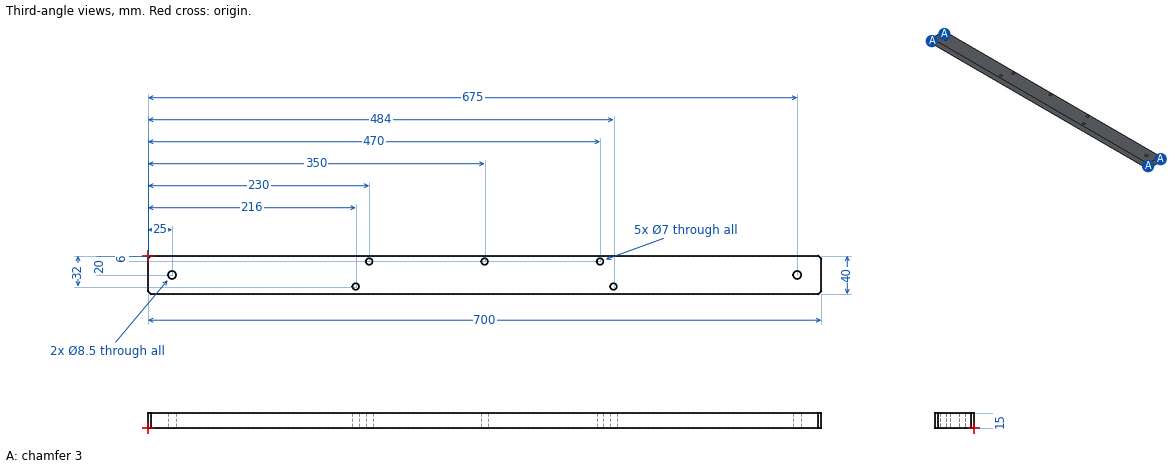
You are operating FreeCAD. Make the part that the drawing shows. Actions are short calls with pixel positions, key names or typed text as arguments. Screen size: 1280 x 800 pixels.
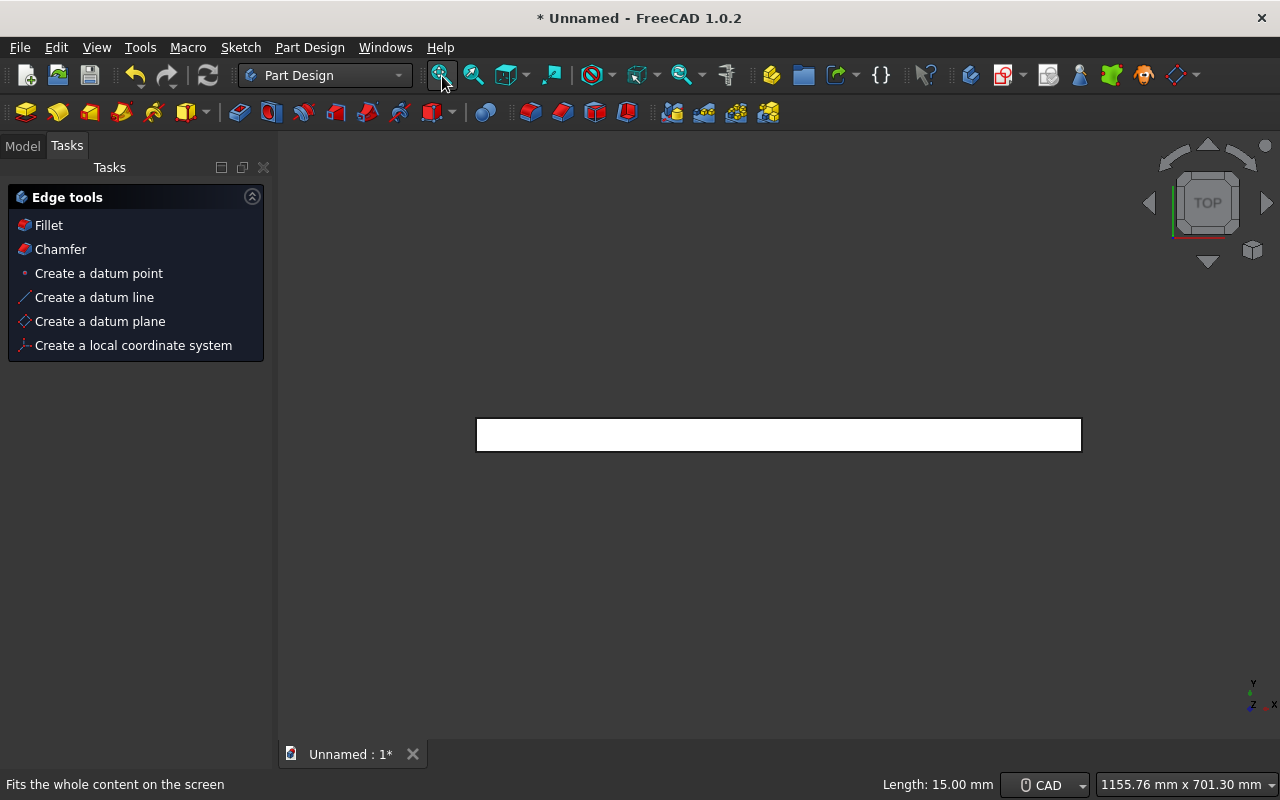
scroll(476, 417, up, 6)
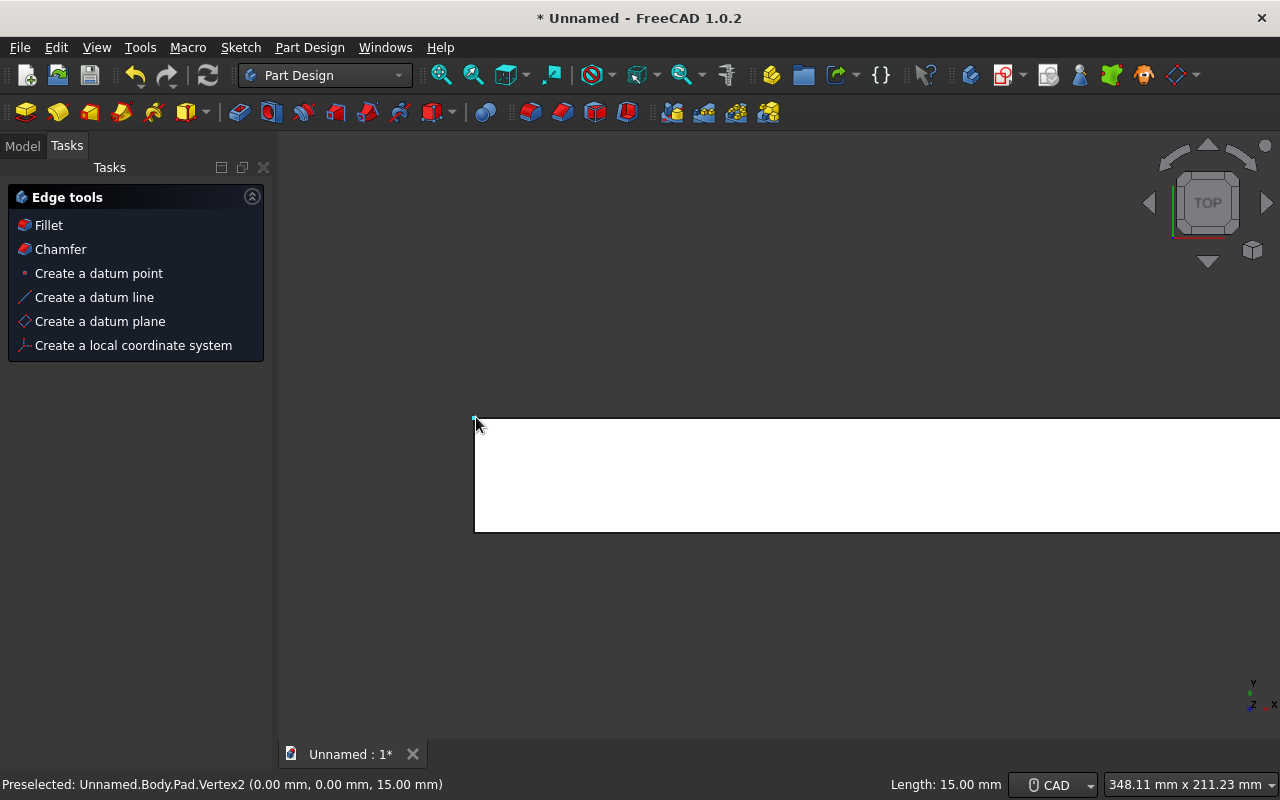
click(442, 76)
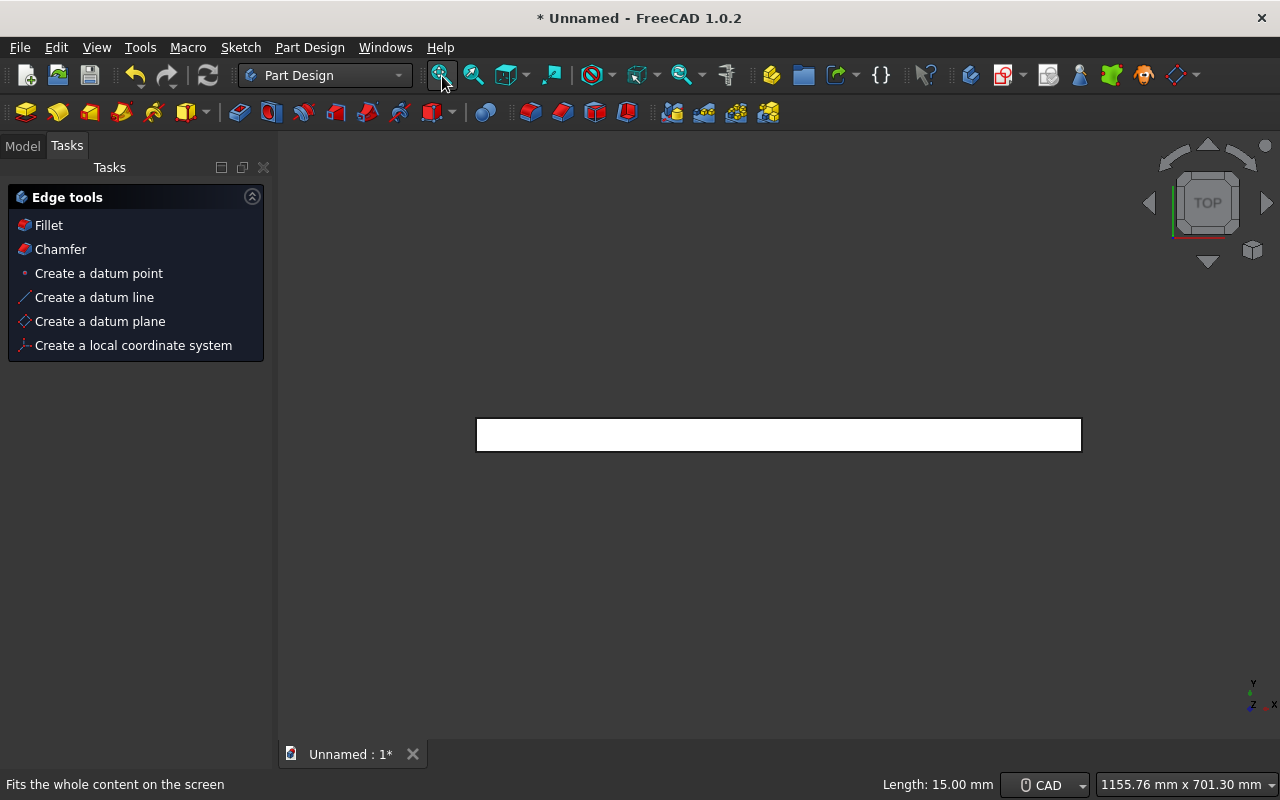
key(1)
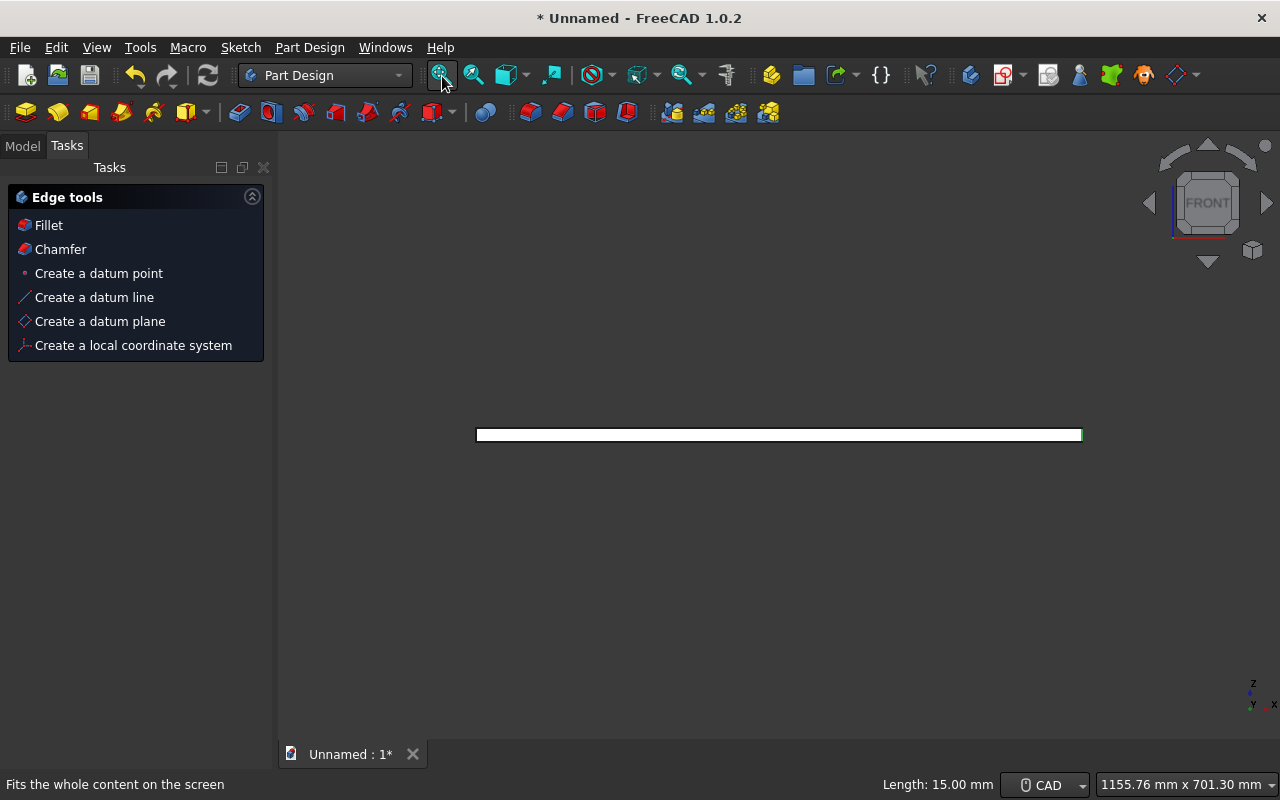
click(476, 434, ctrl)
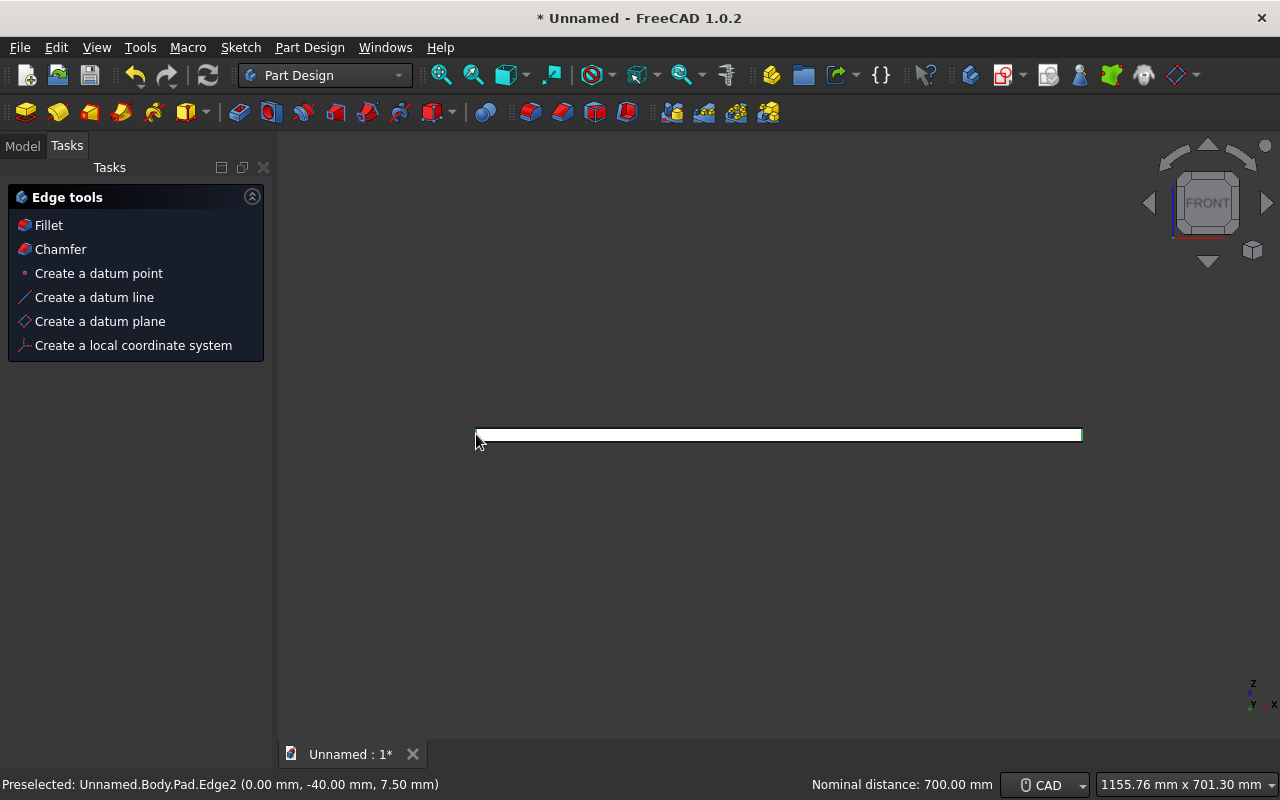
scroll(476, 434, up, 6)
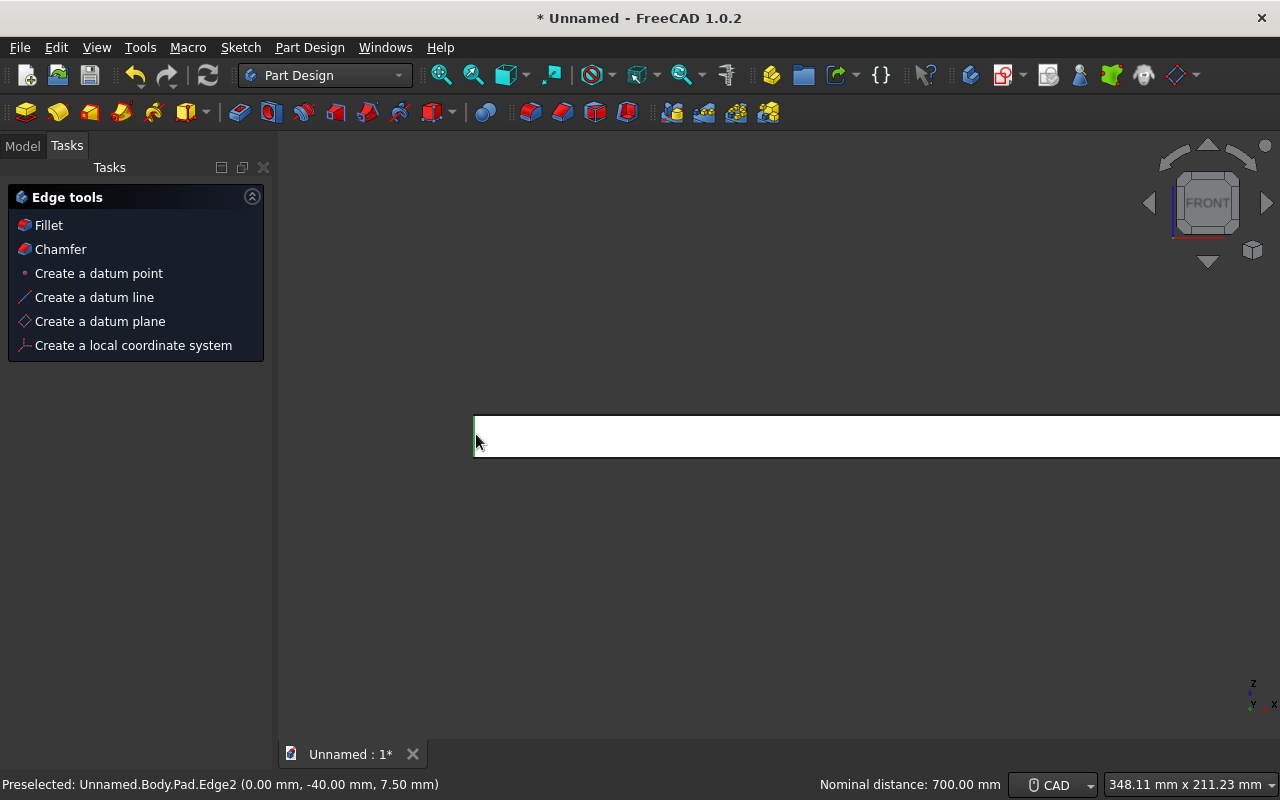
click(442, 76)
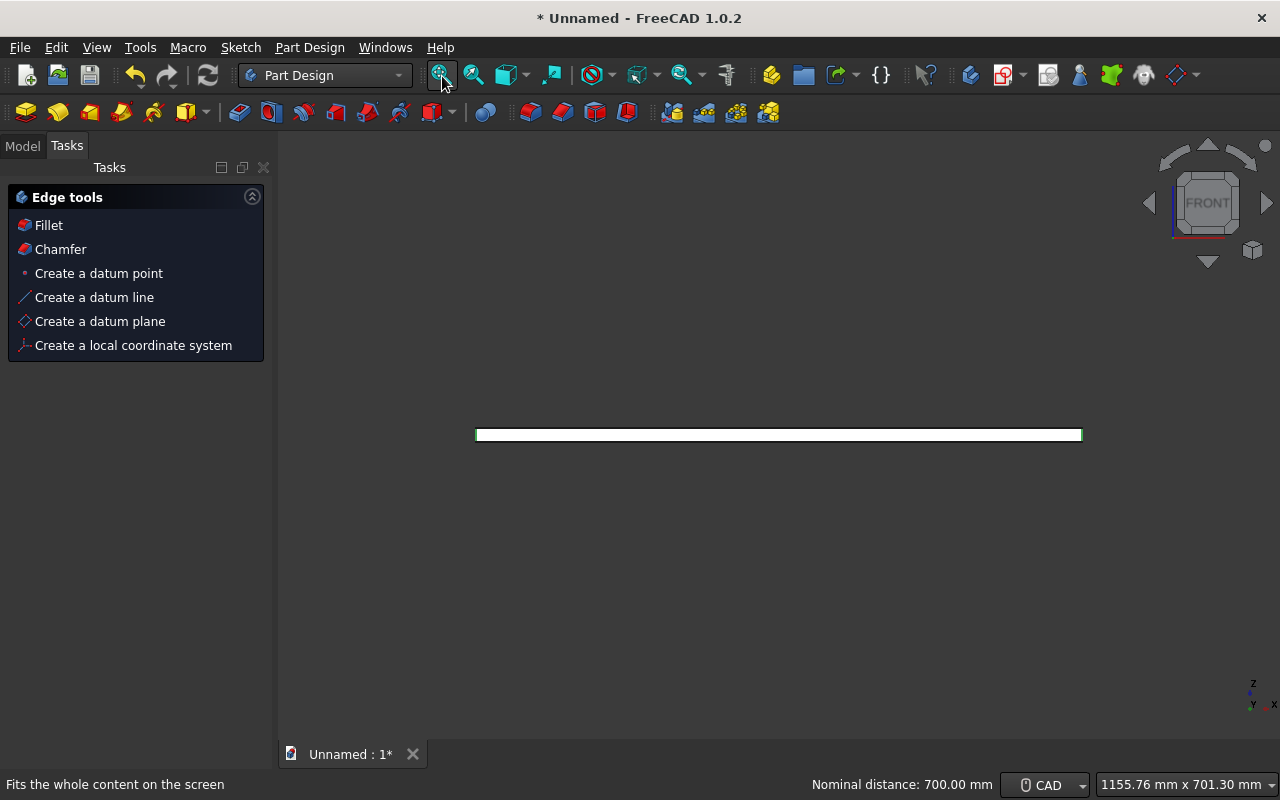
key(3)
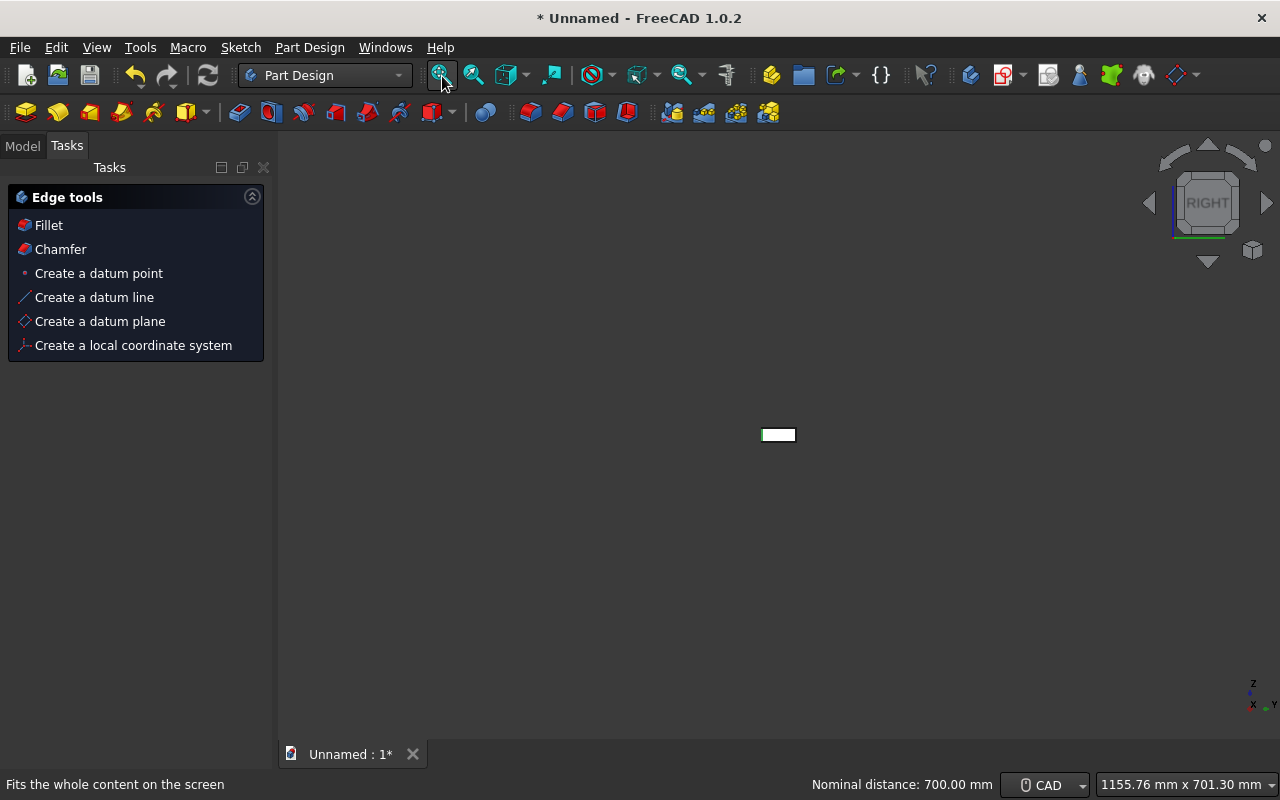
click(442, 76)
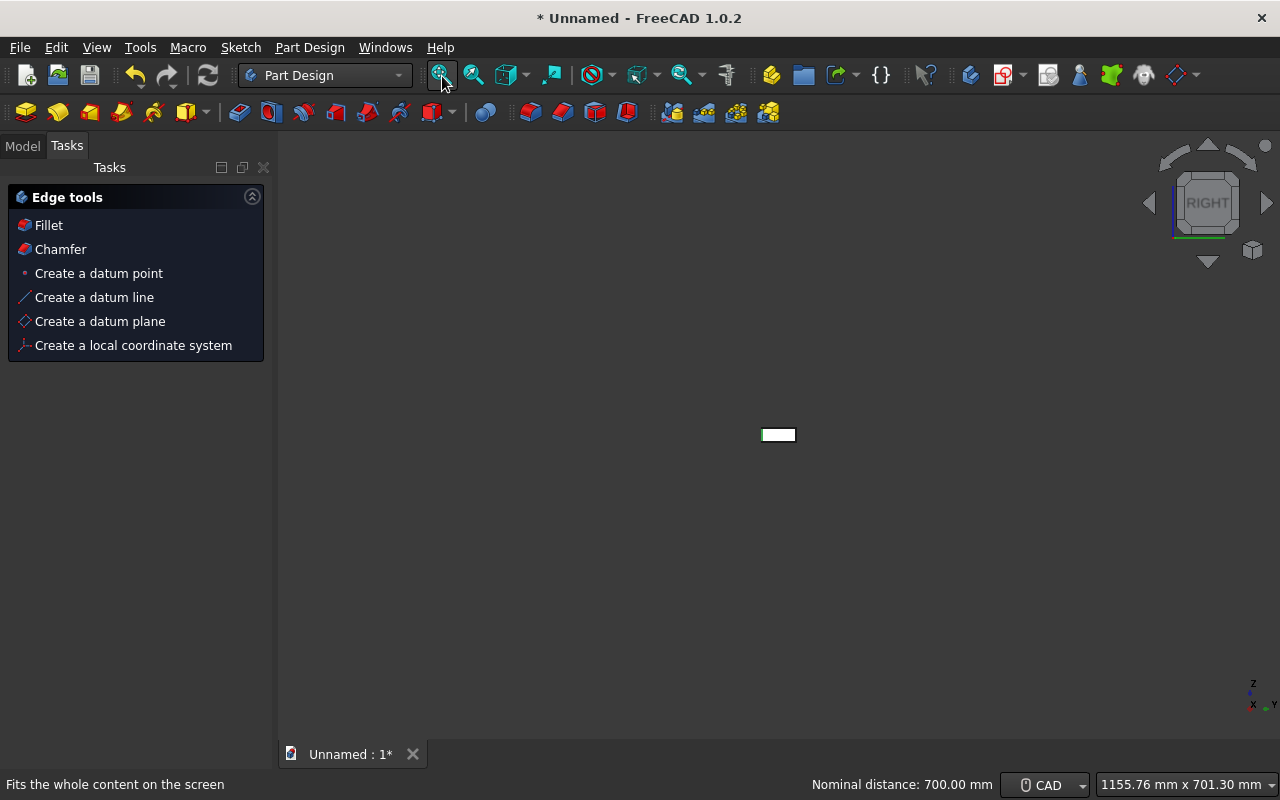
click(796, 434, ctrl)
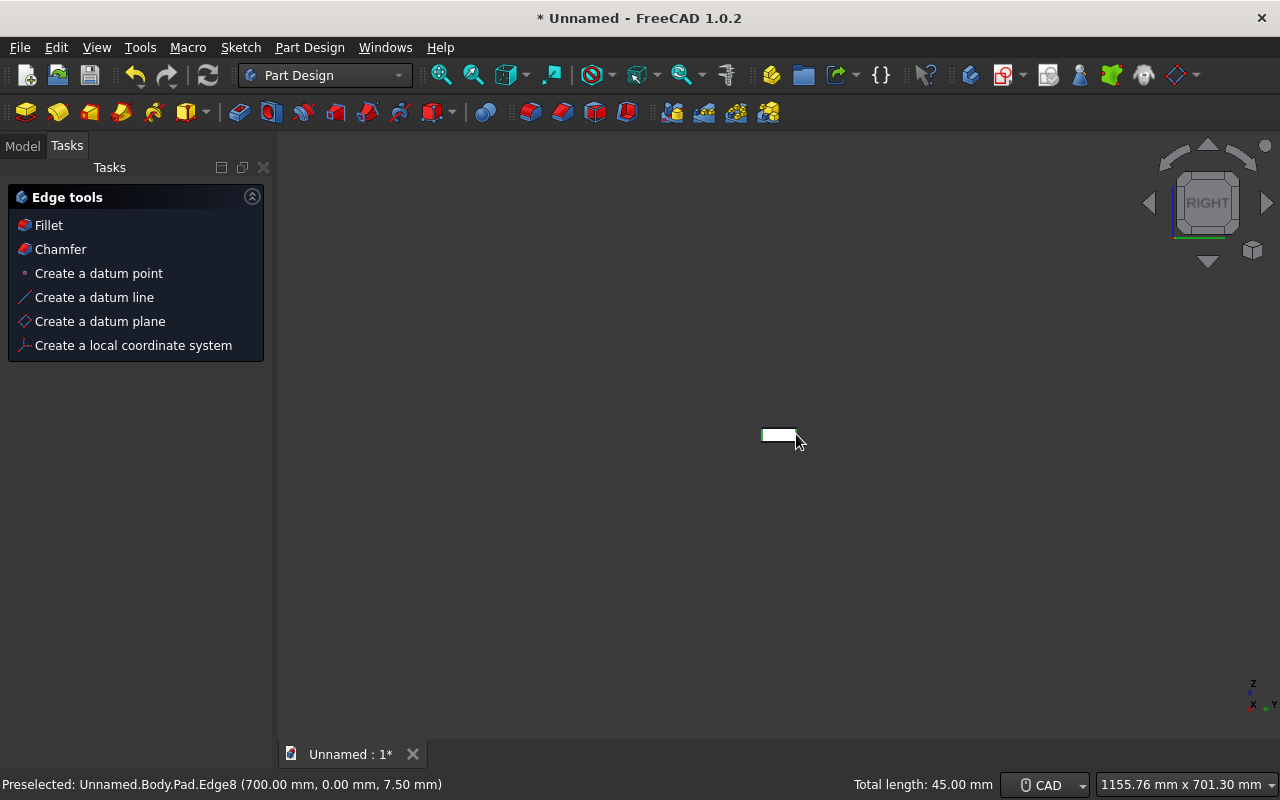
scroll(796, 434, up, 6)